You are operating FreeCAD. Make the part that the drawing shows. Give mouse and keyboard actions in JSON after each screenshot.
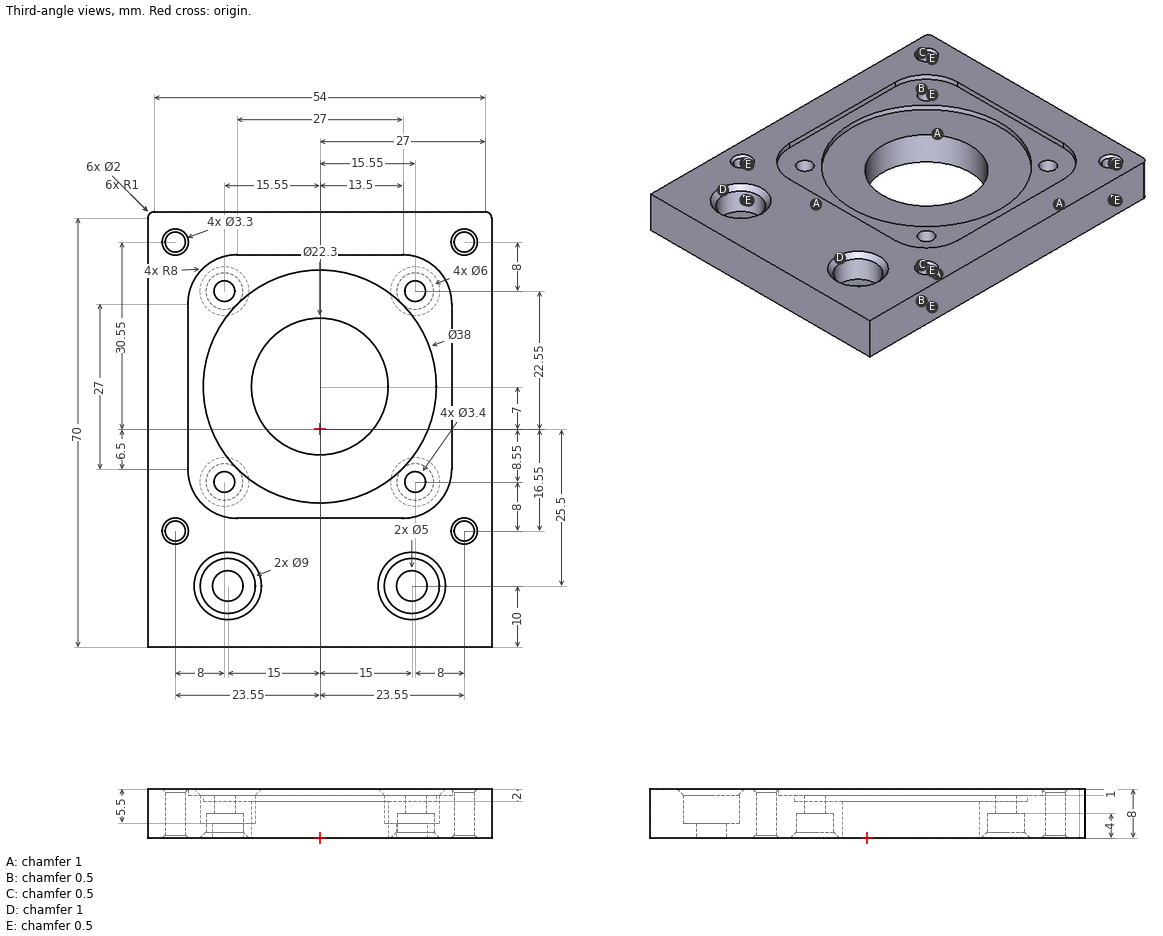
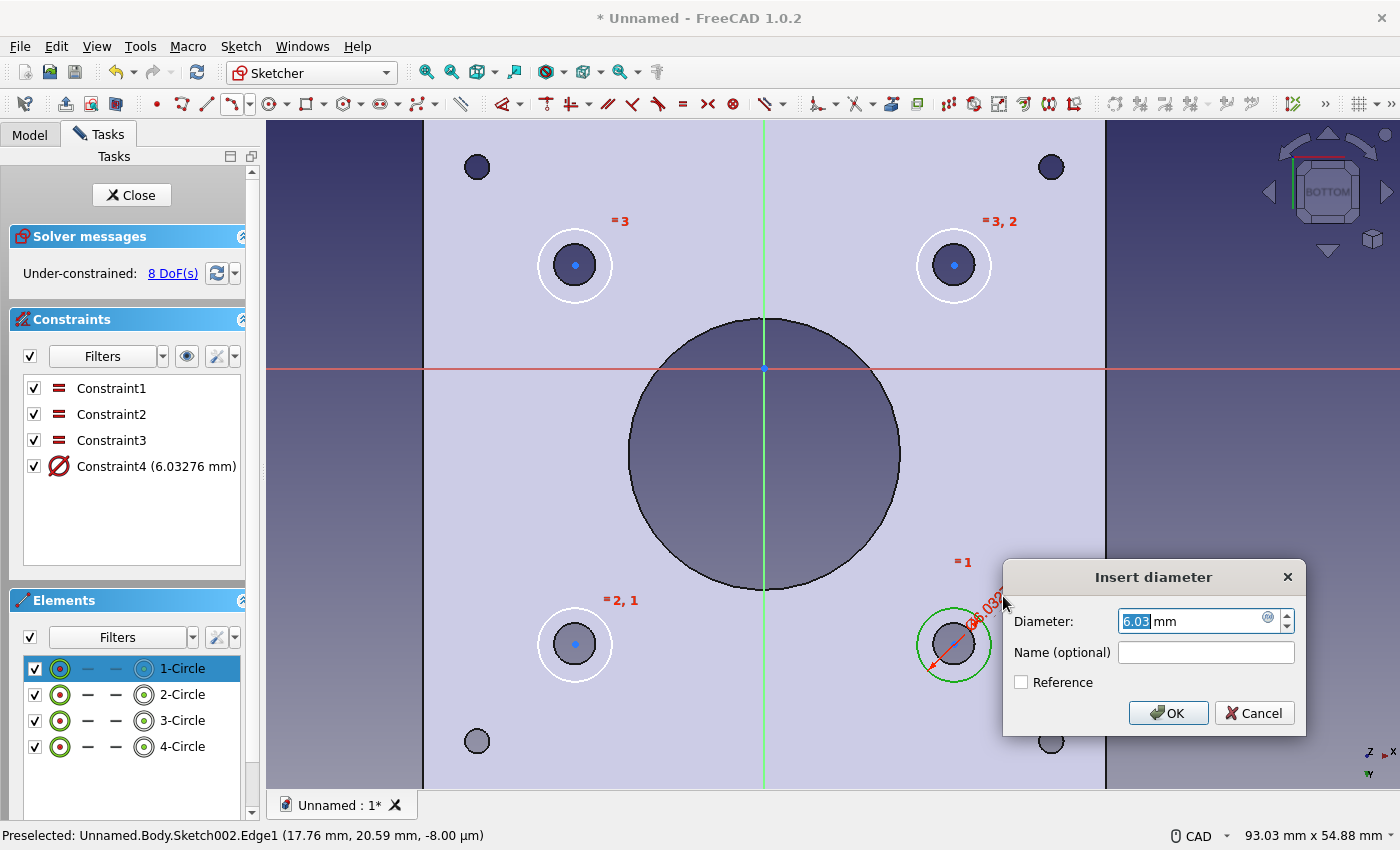
{"action": "type", "text": "6"}
{"action": "key", "text": "Return"}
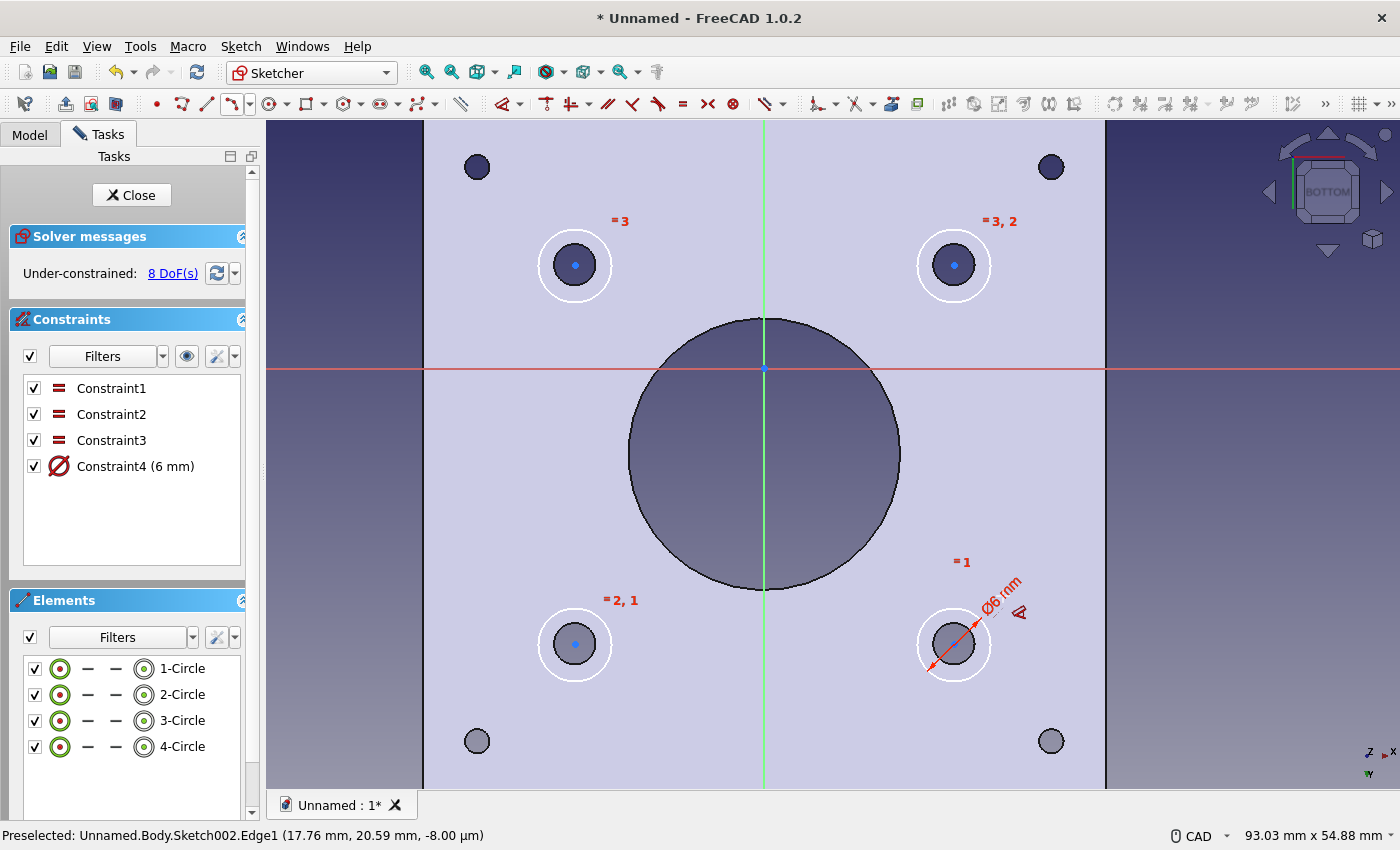
{"action": "left_click", "coordinate": [954, 266]}
{"action": "left_click", "coordinate": [988, 317]}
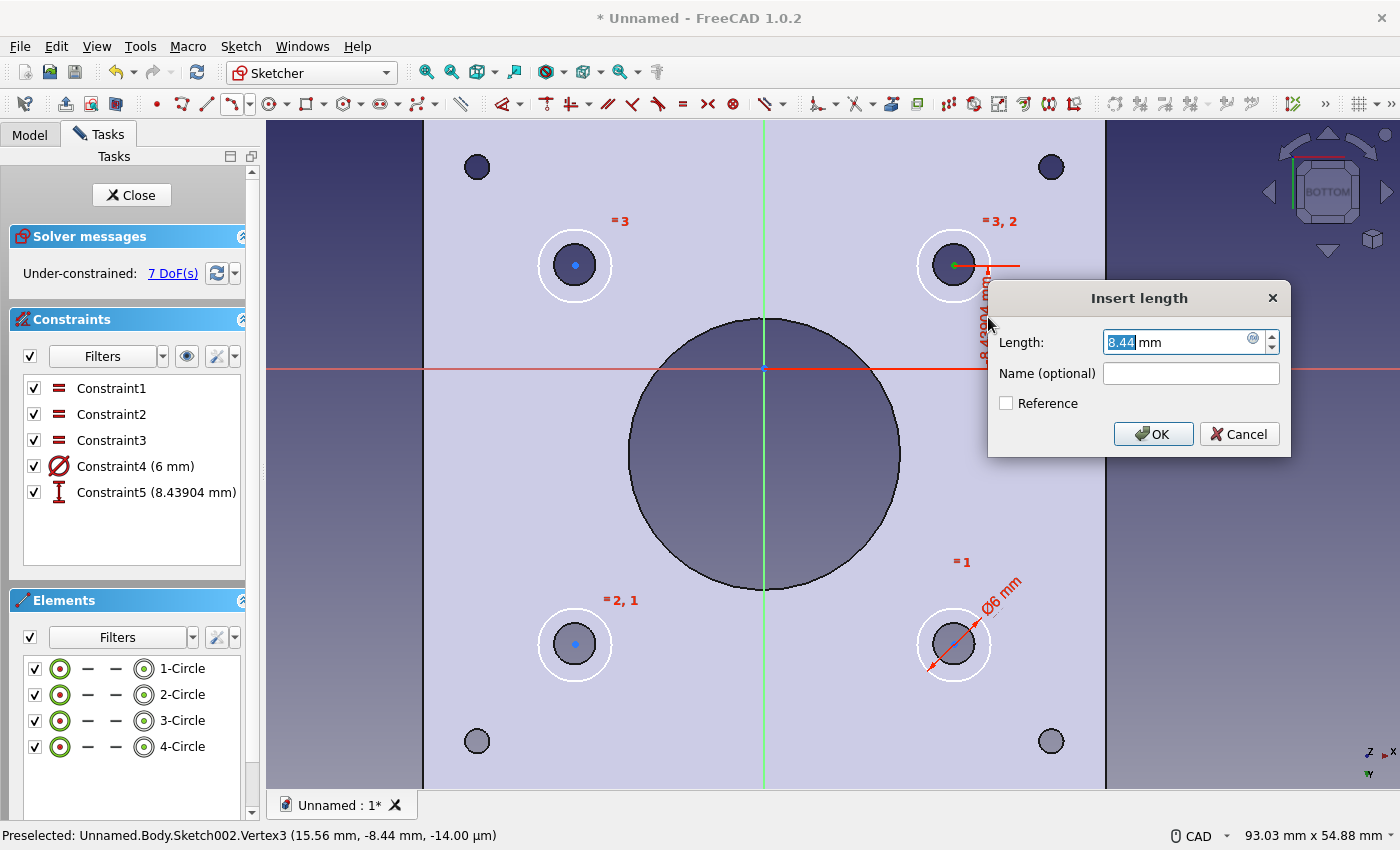
{"action": "type", "text": "8.55"}
{"action": "key", "text": "Return"}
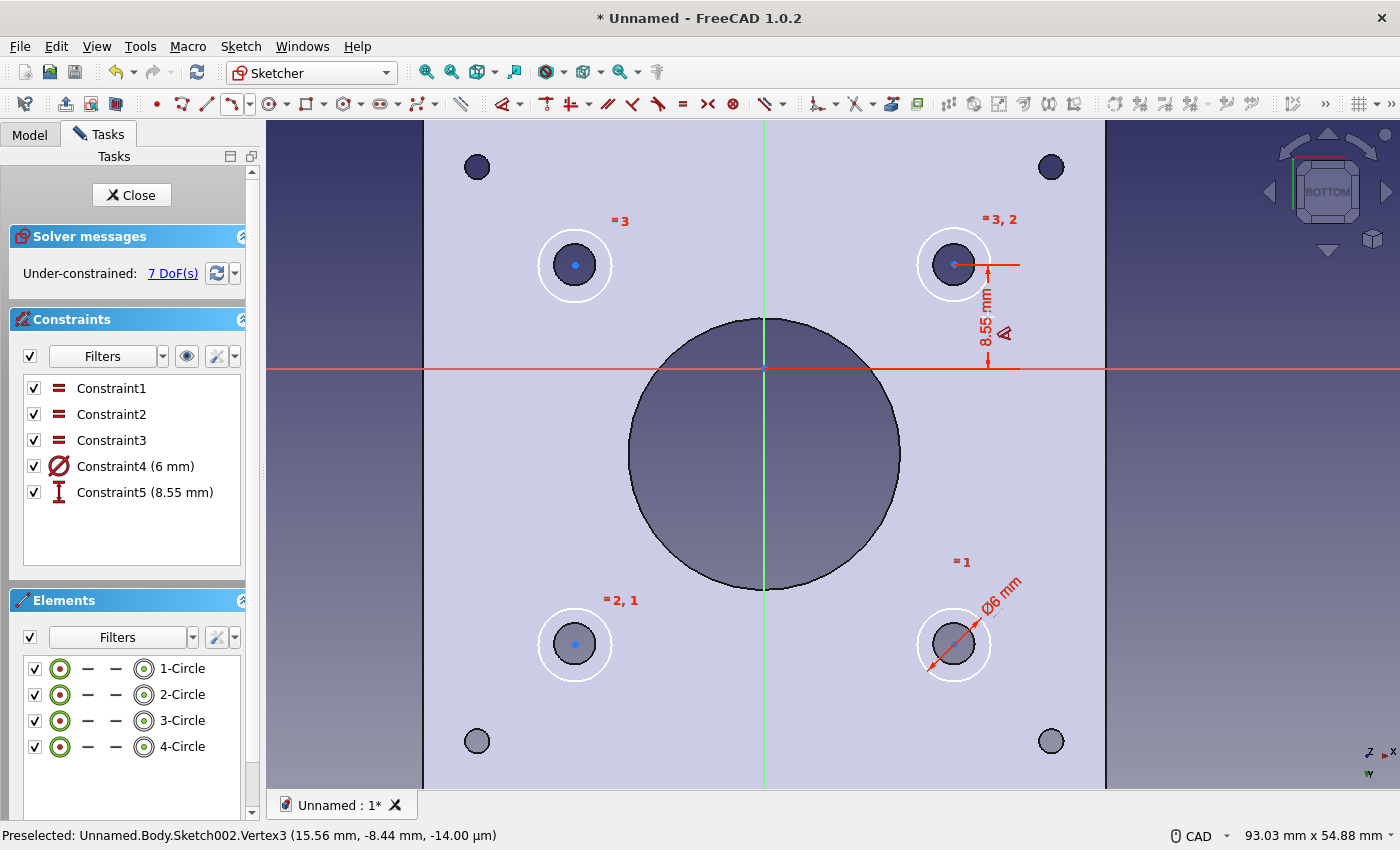
{"action": "left_click", "coordinate": [575, 266]}
{"action": "left_click", "coordinate": [541, 317]}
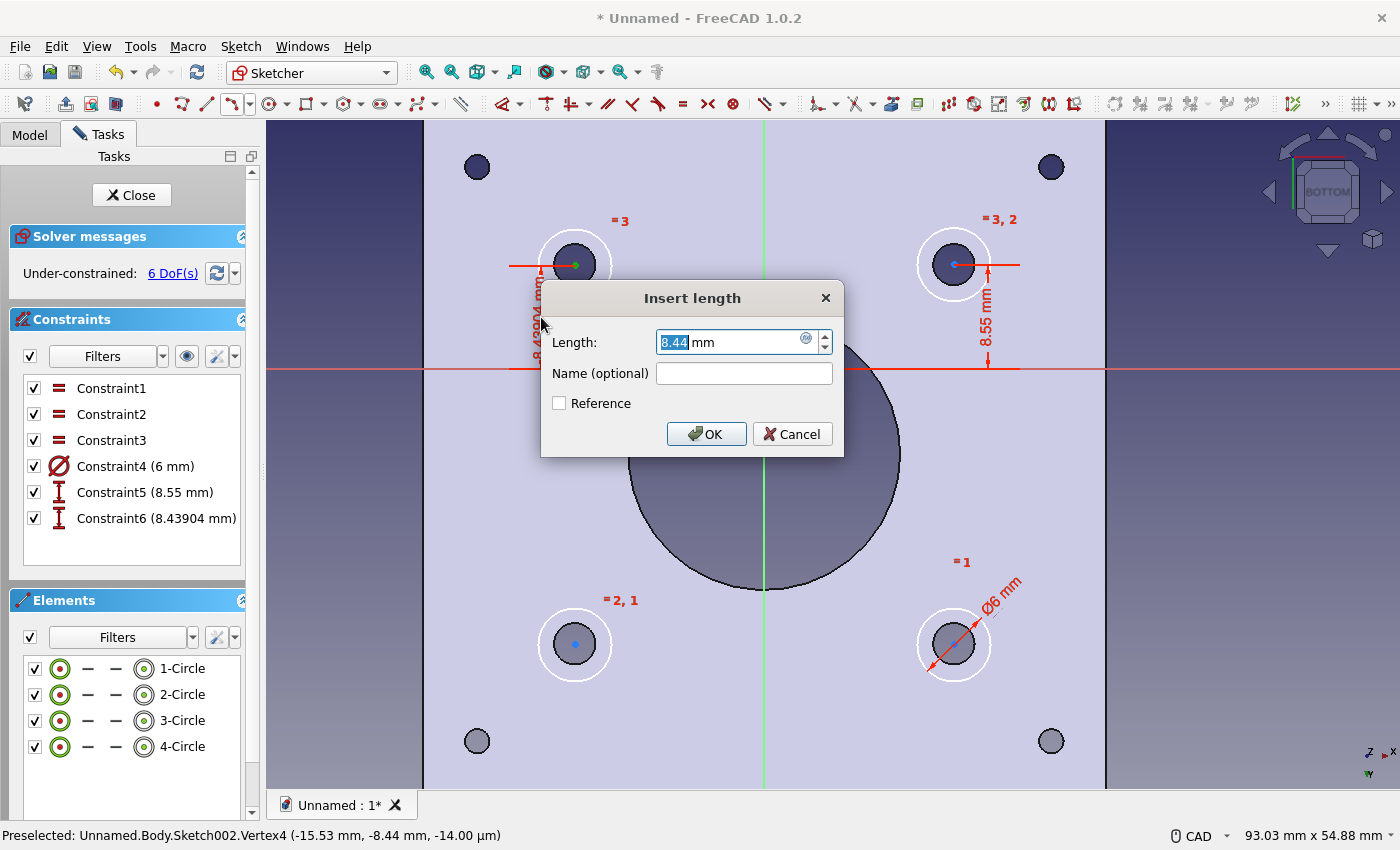
{"action": "type", "text": "8.55"}
{"action": "key", "text": "Return"}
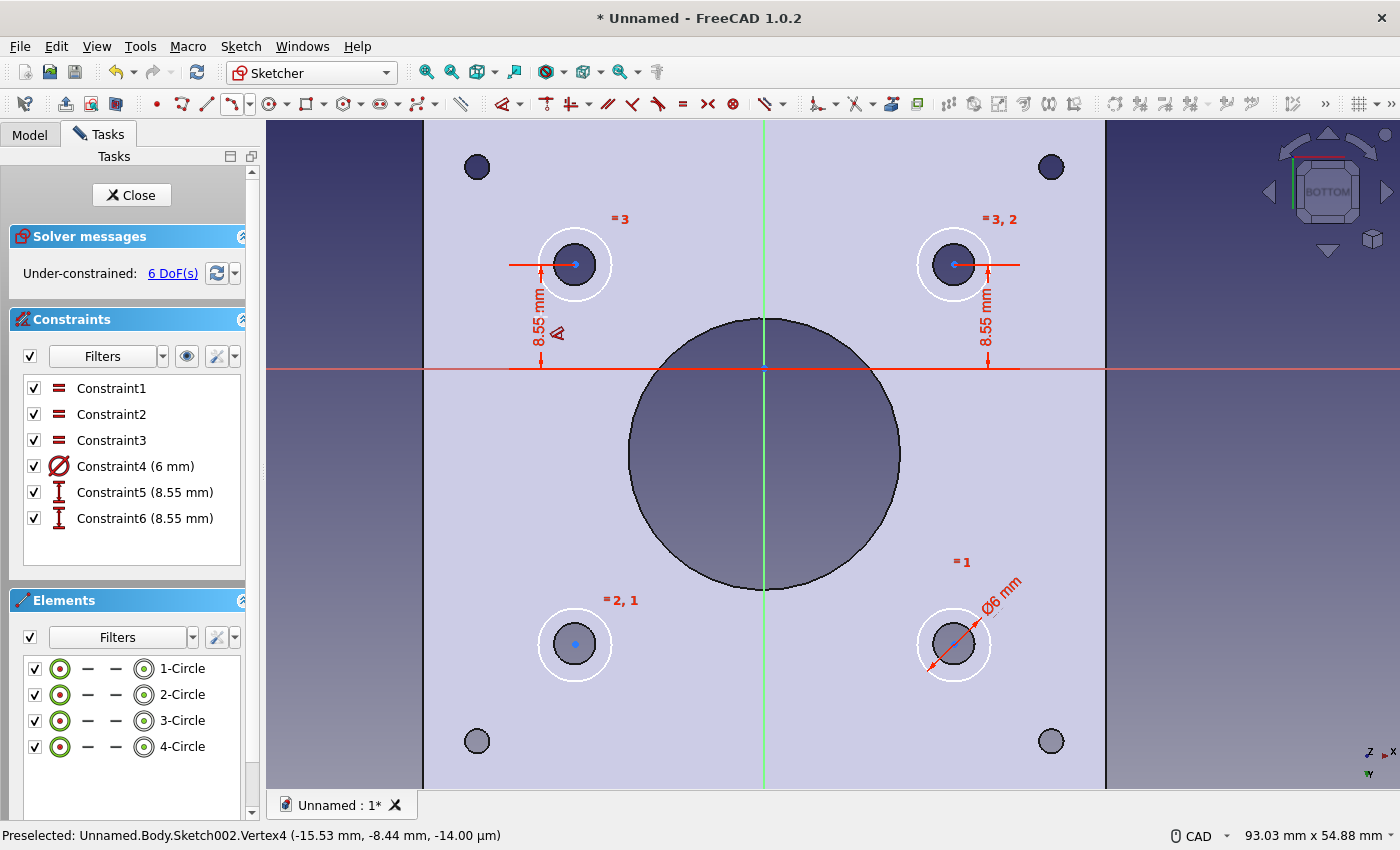
{"action": "left_click", "coordinate": [954, 645]}
{"action": "left_click", "coordinate": [859, 679]}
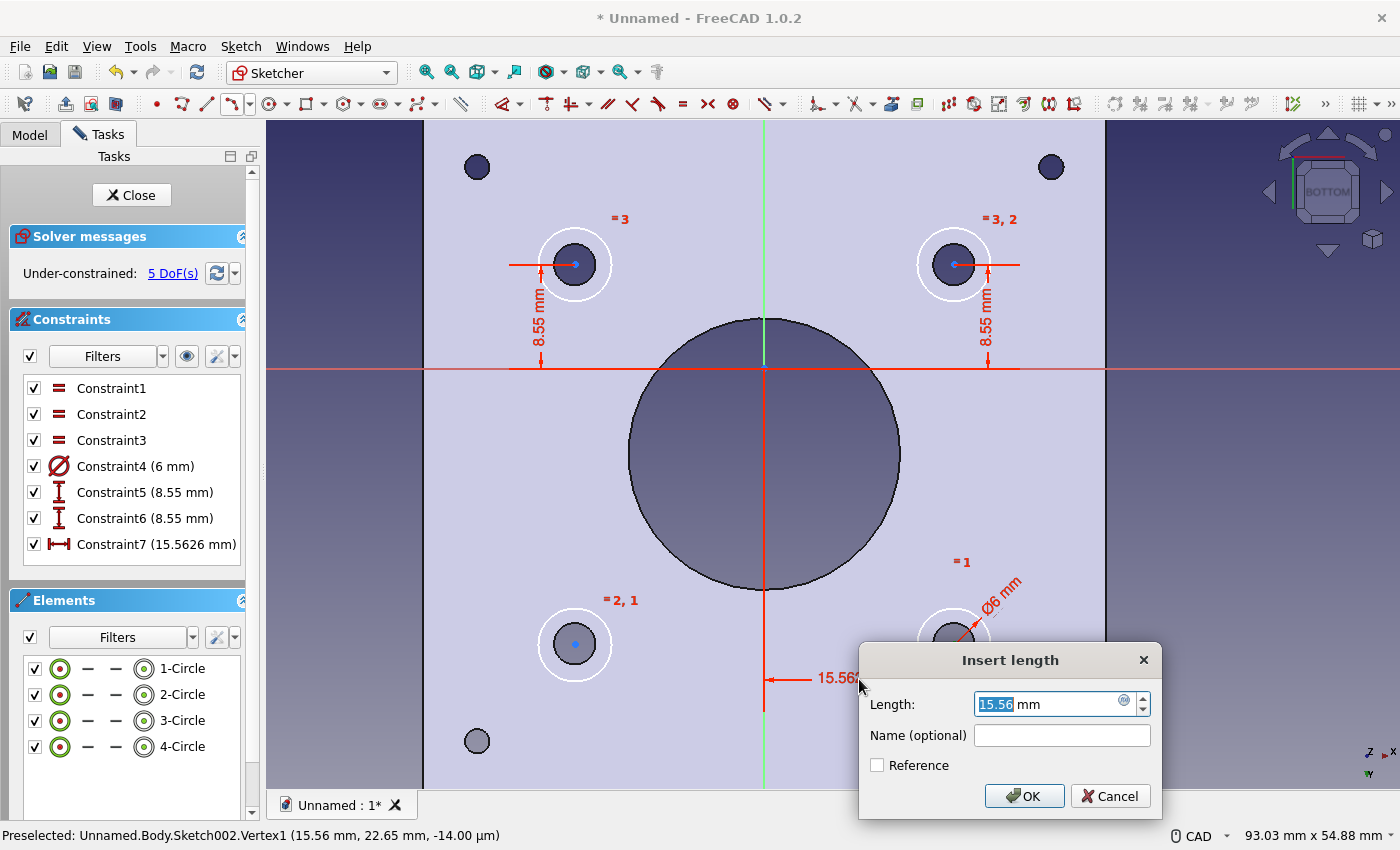
{"action": "type", "text": "15.55"}
{"action": "key", "text": "Return"}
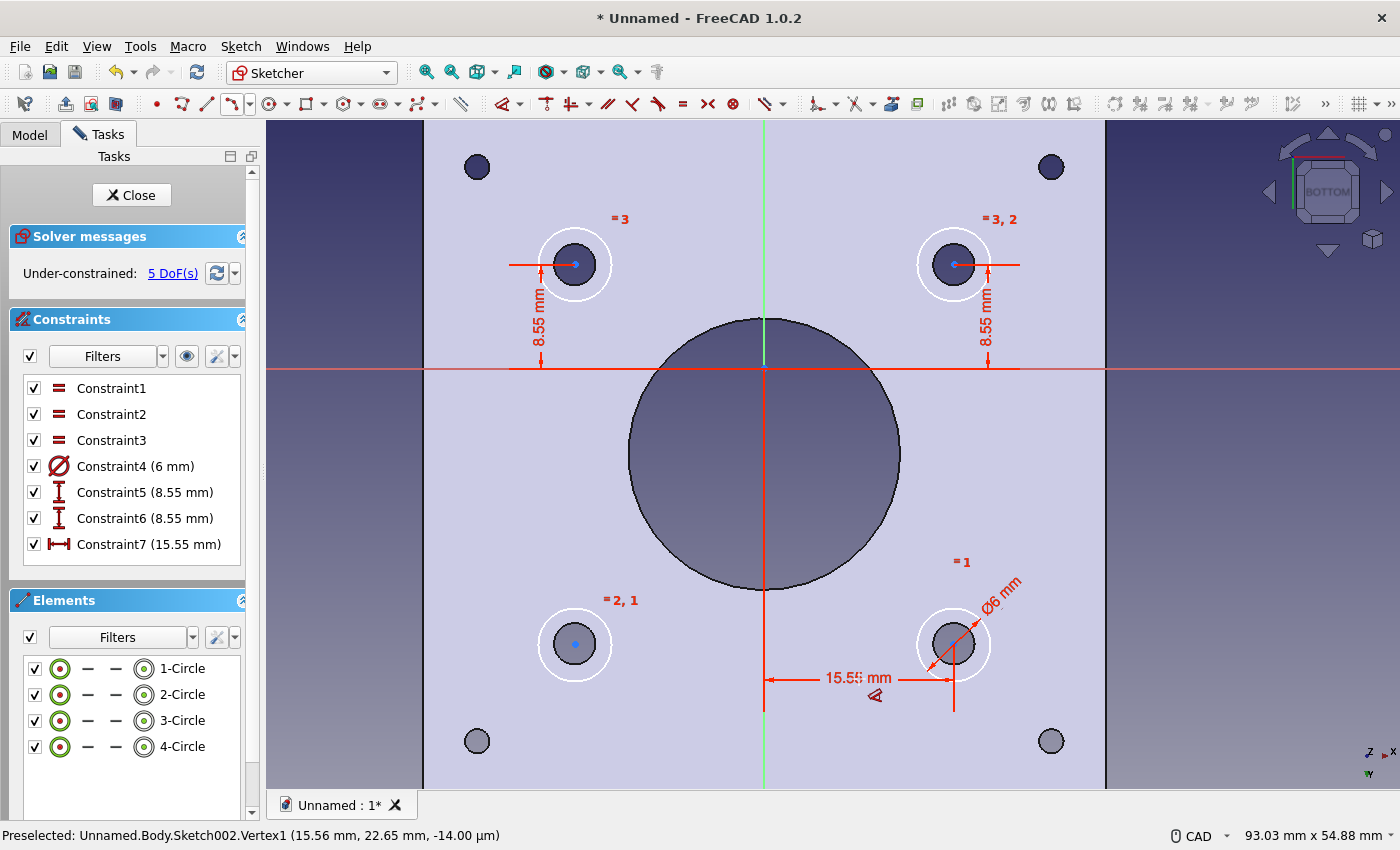
{"action": "left_click", "coordinate": [954, 645]}
{"action": "left_click", "coordinate": [988, 507]}